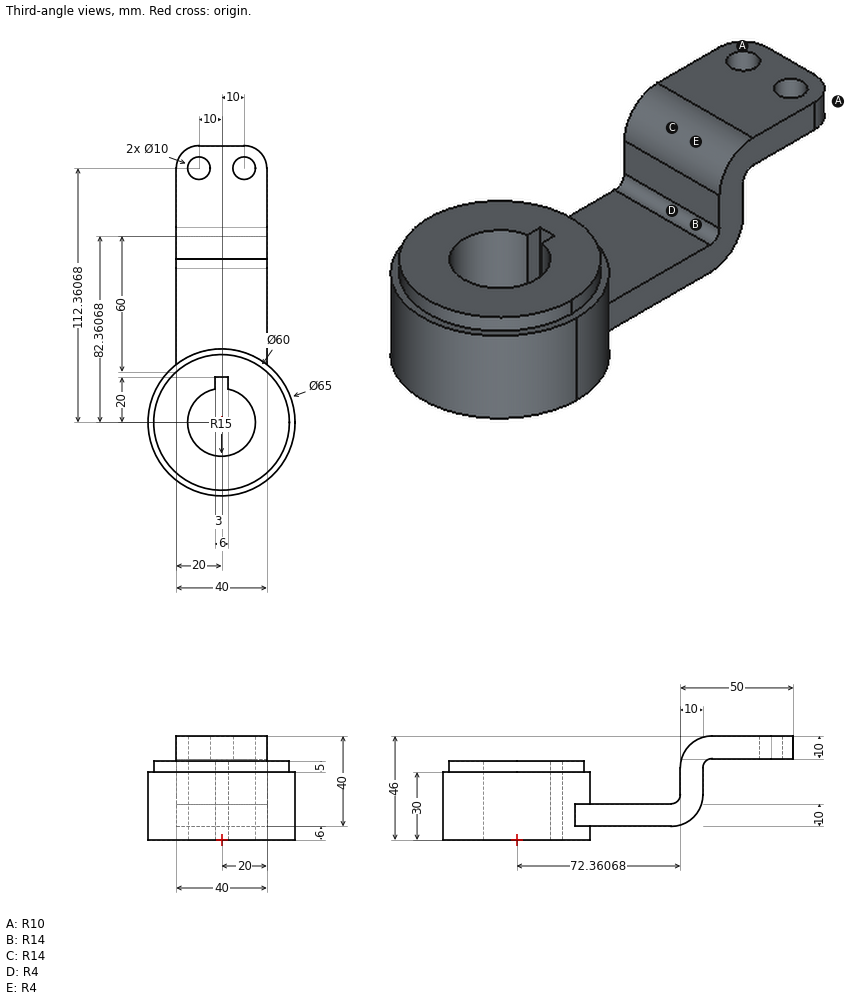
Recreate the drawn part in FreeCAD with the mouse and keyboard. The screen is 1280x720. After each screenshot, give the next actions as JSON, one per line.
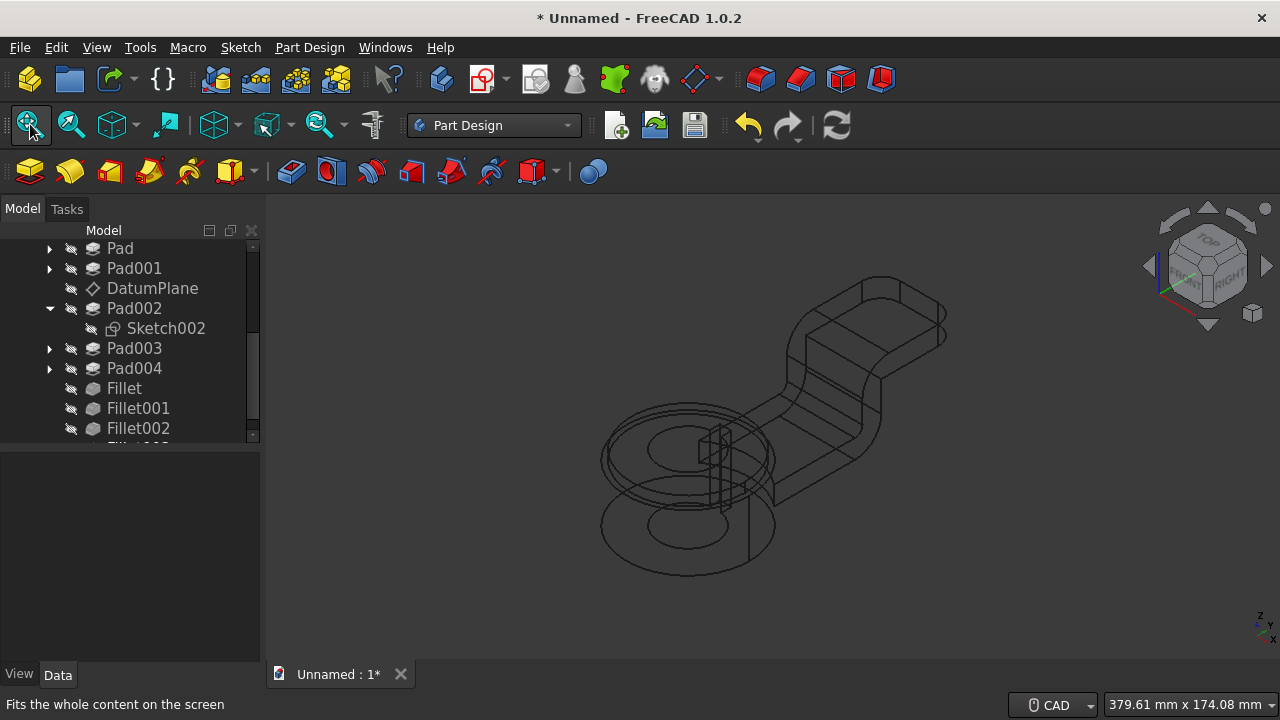
{"action": "left_click", "coordinate": [844, 356]}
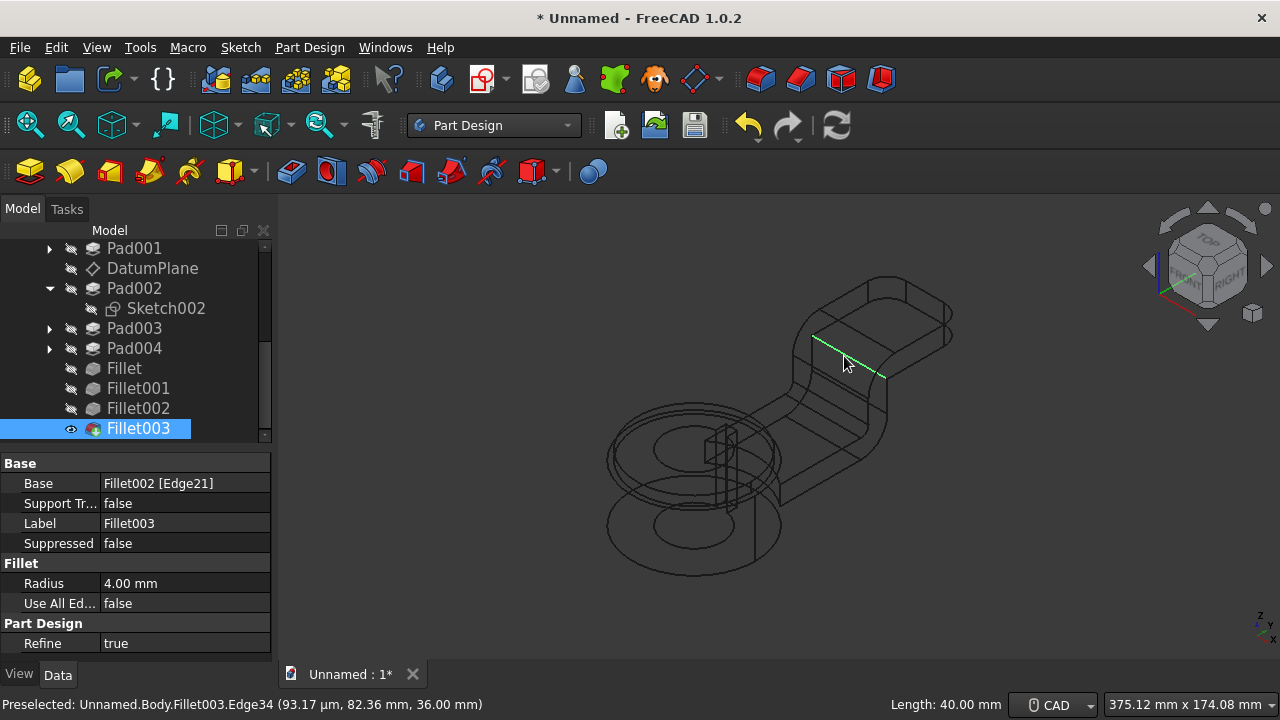
{"action": "key", "text": "v 1"}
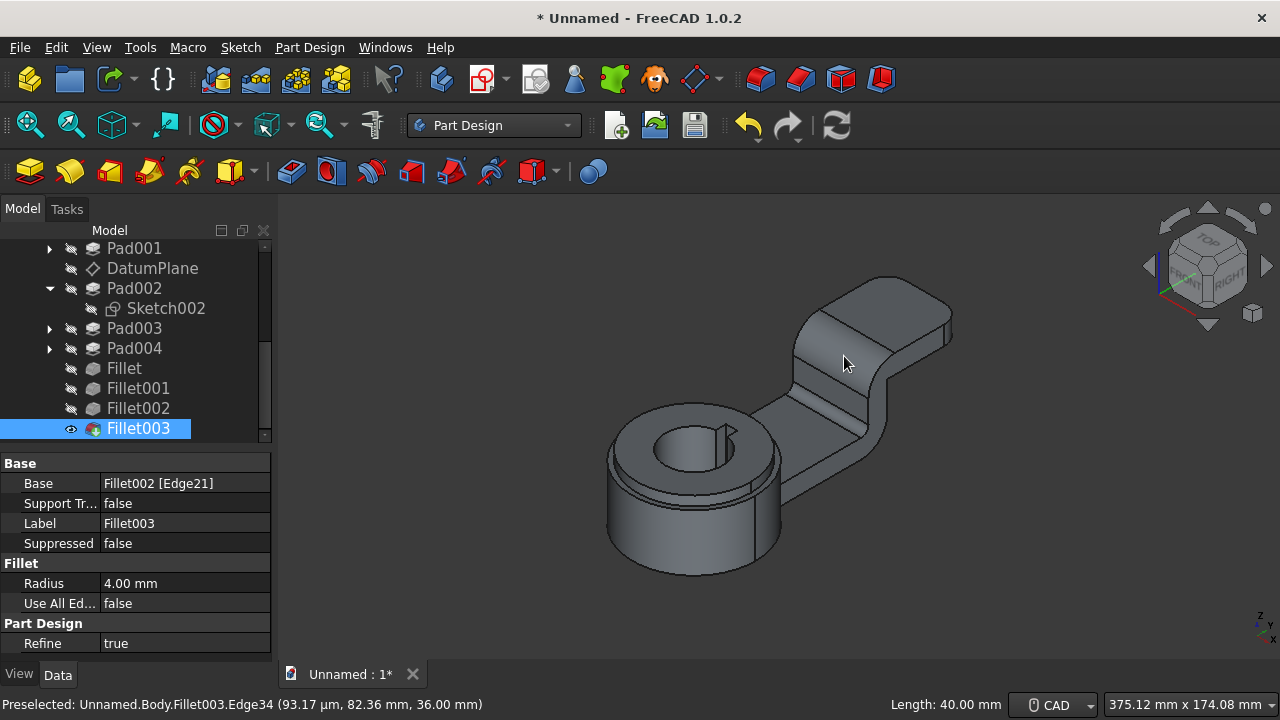
{"action": "left_click", "coordinate": [762, 80]}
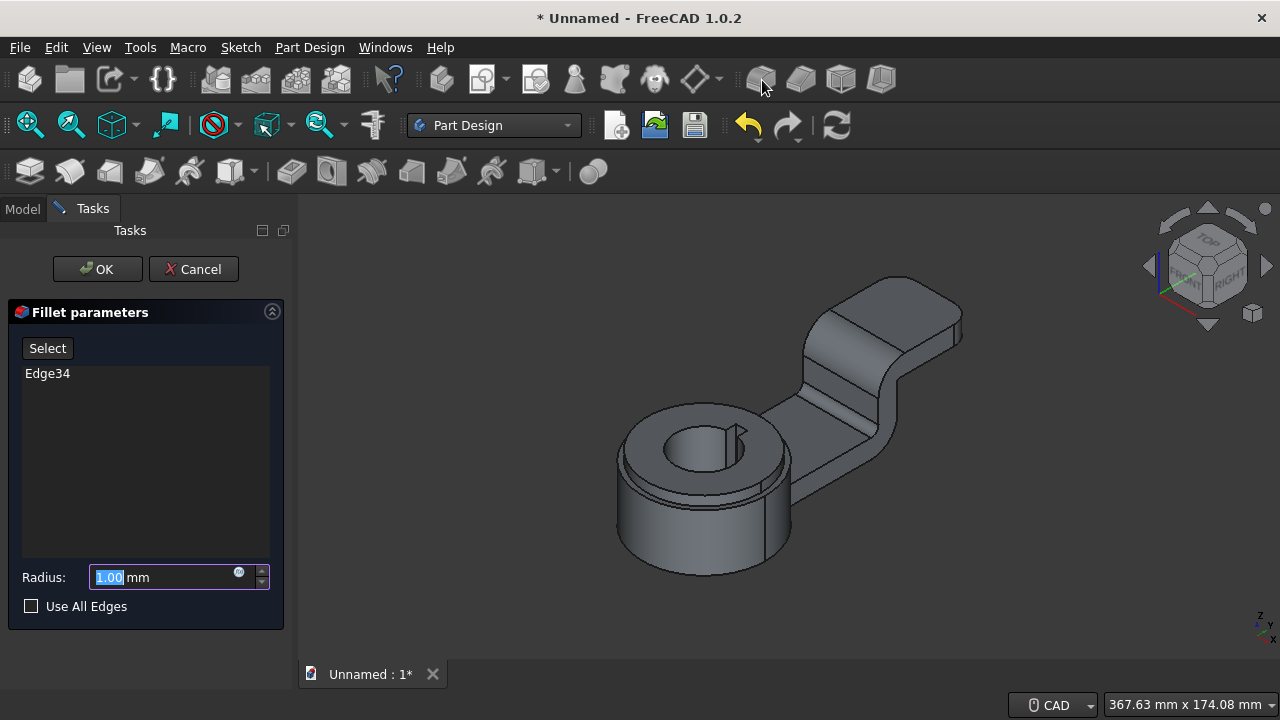
{"action": "type", "text": "4"}
{"action": "key", "text": "Tab"}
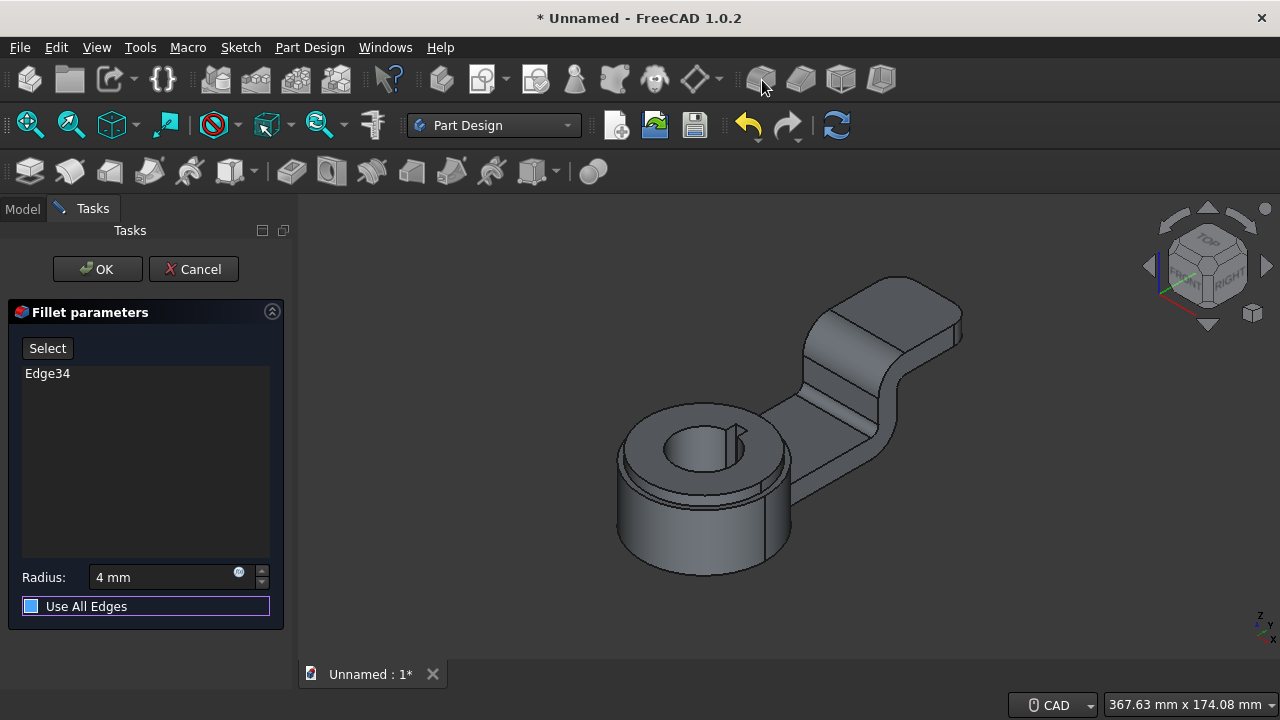
{"action": "left_click", "coordinate": [98, 269]}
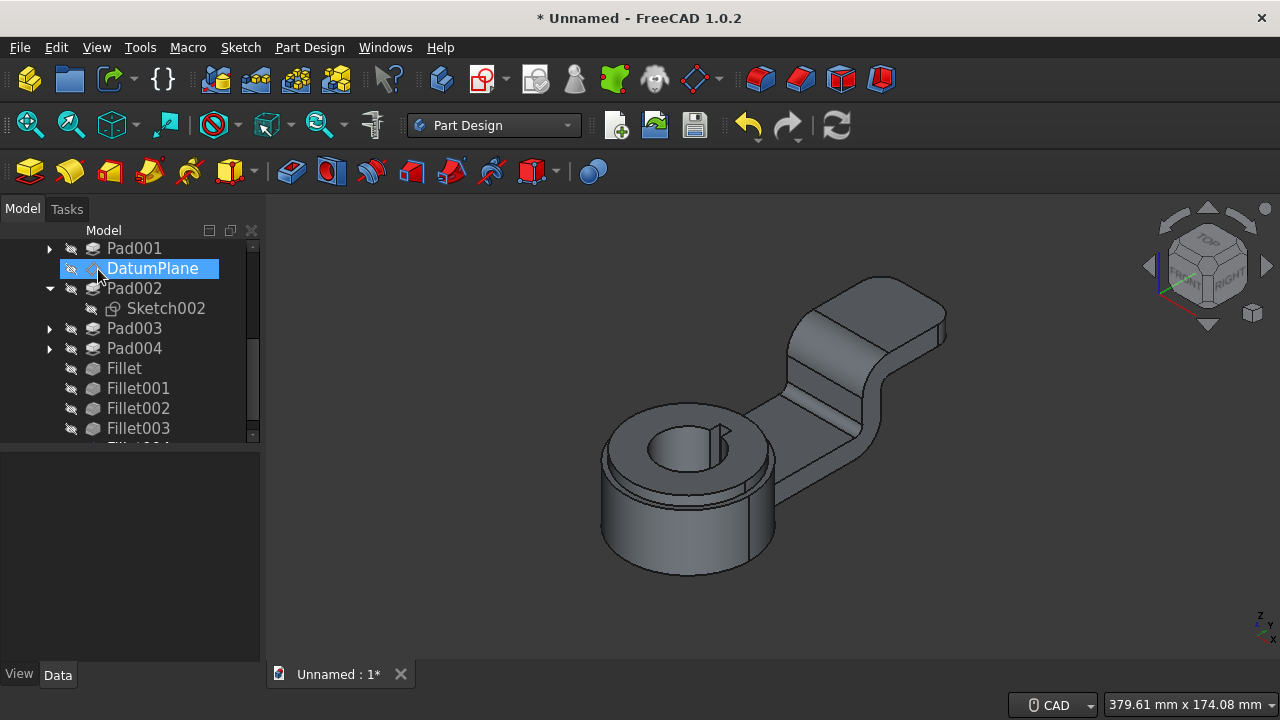
{"action": "left_click", "coordinate": [885, 310]}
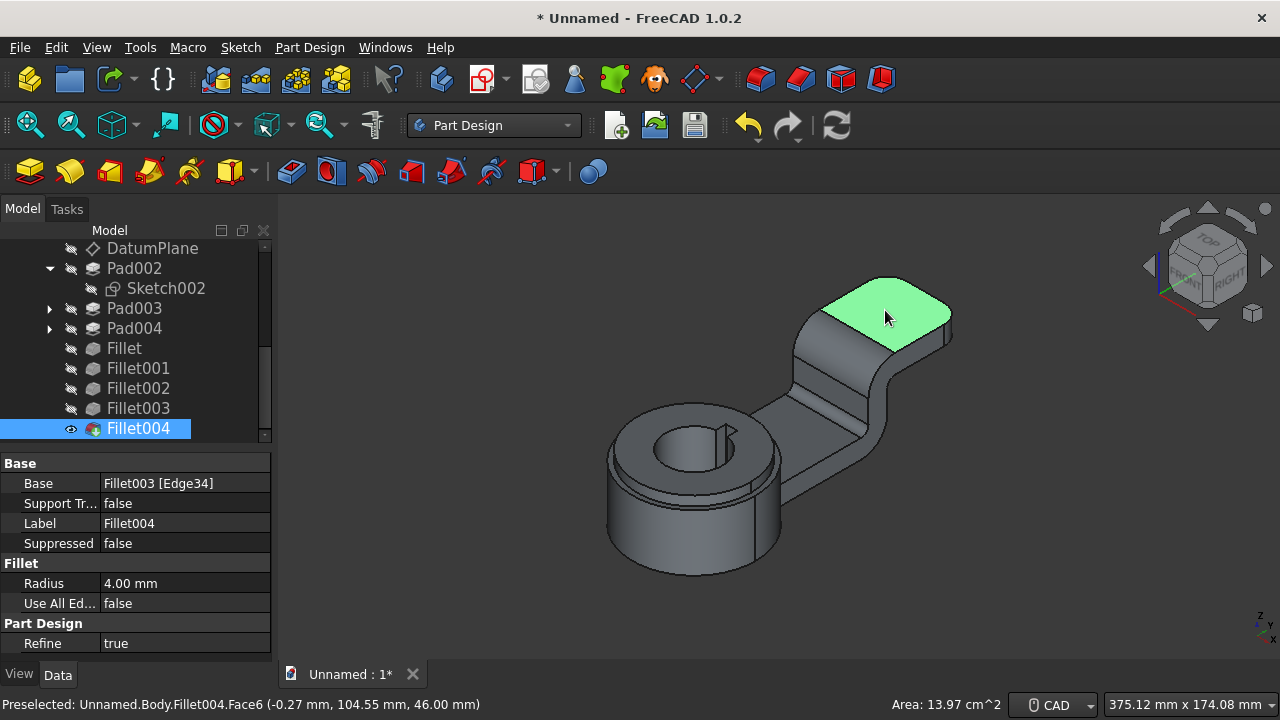
{"action": "left_click", "coordinate": [482, 80]}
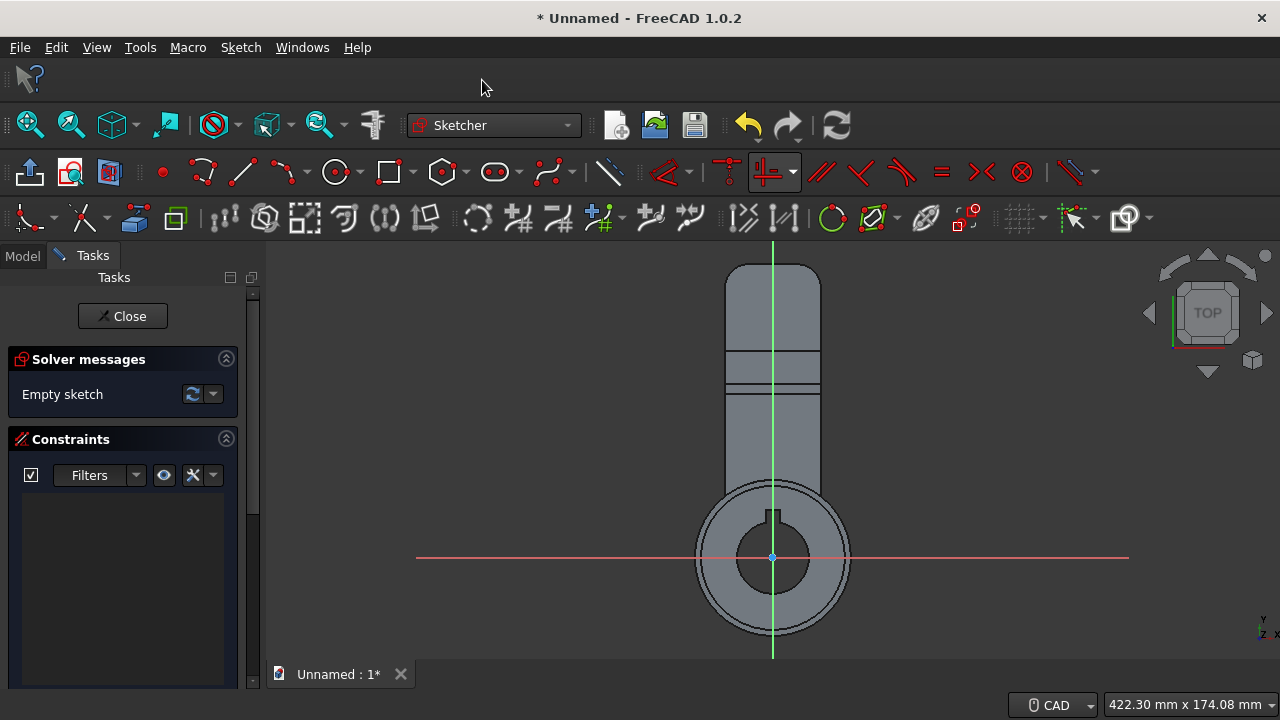
{"action": "scroll", "coordinate": [784, 269], "scroll_direction": "up", "scroll_amount": 10}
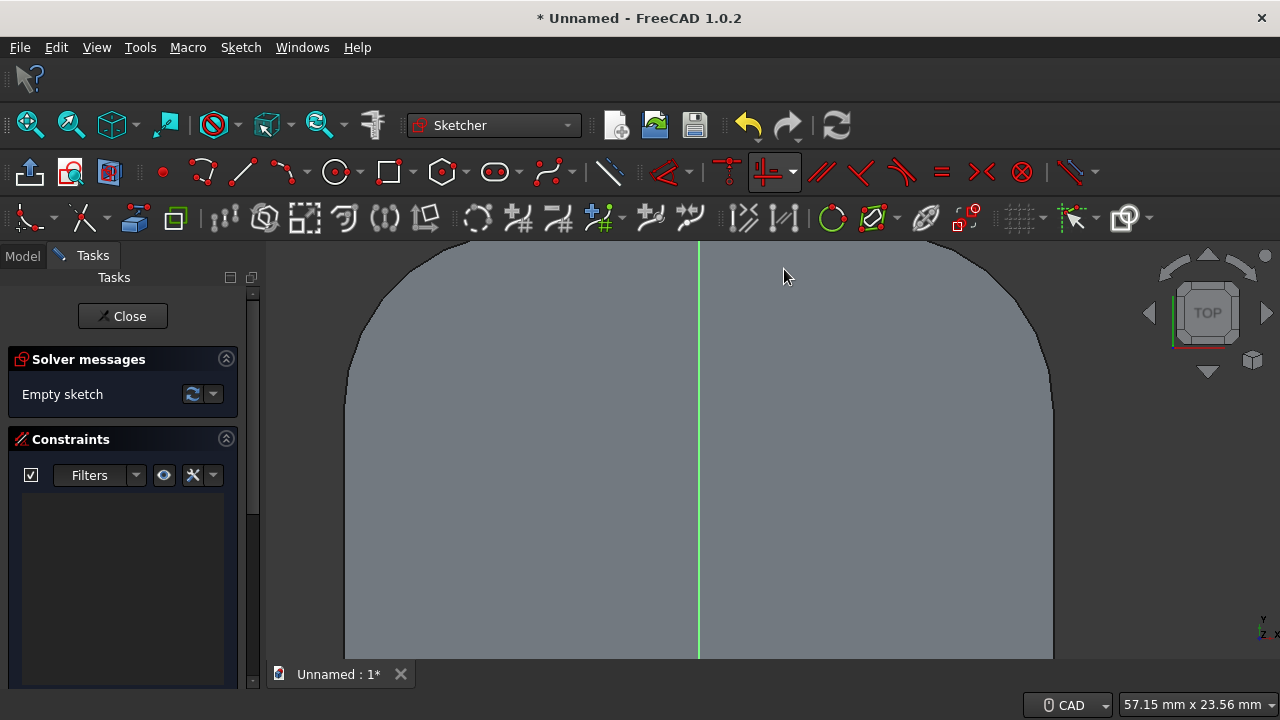
{"action": "key", "text": "g c"}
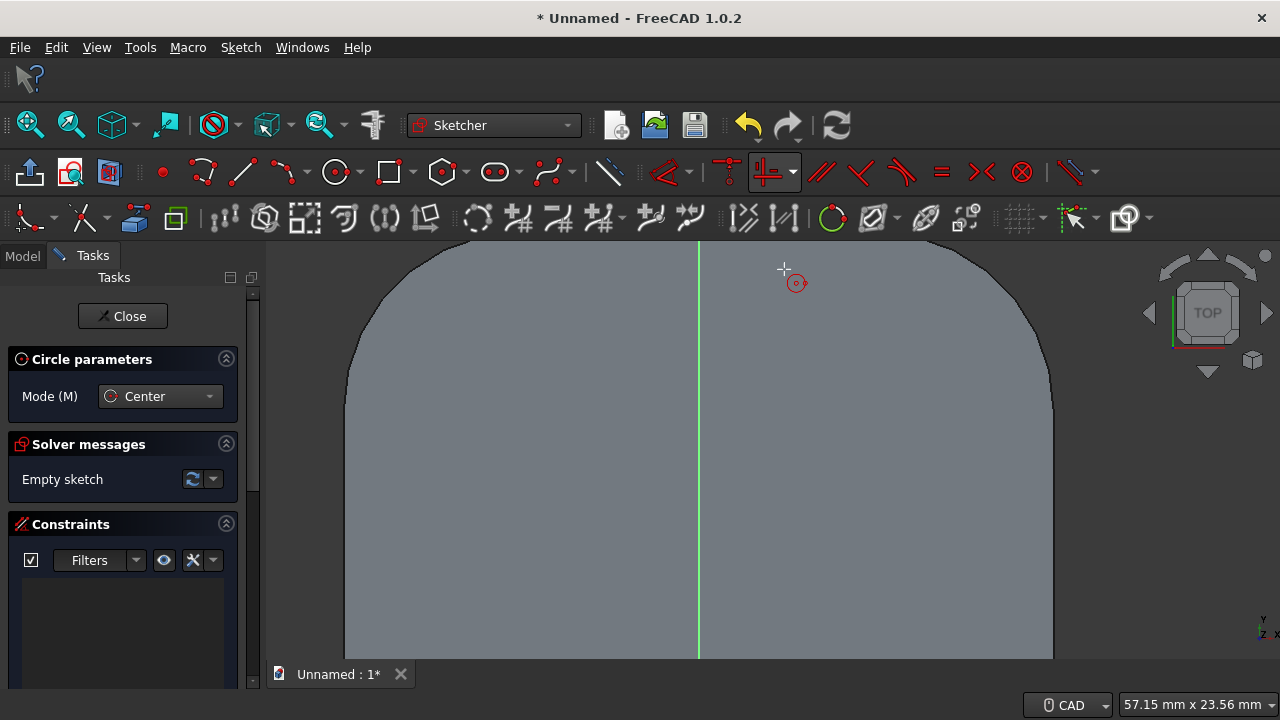
{"action": "left_click", "coordinate": [521, 410]}
{"action": "left_click", "coordinate": [584, 347]}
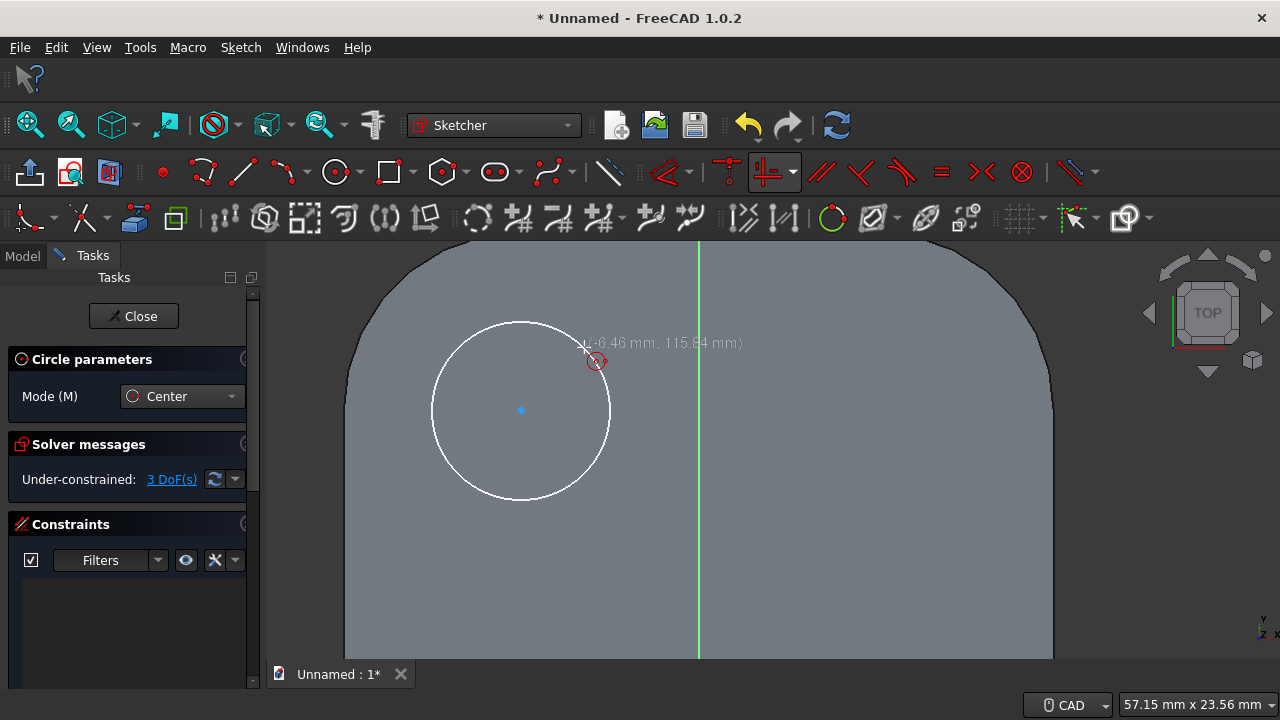
{"action": "left_click", "coordinate": [876, 410]}
{"action": "left_click", "coordinate": [939, 347]}
{"action": "key", "text": "Escape"}